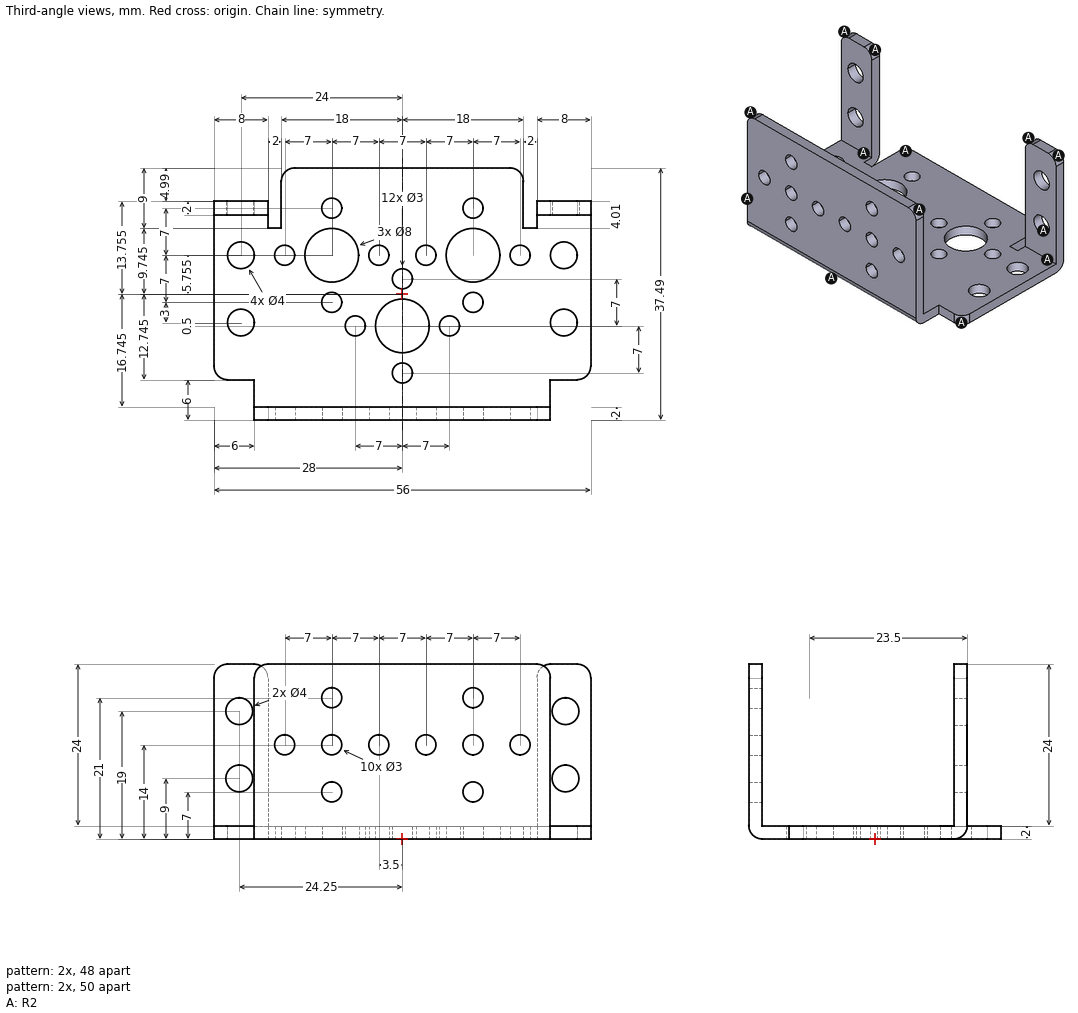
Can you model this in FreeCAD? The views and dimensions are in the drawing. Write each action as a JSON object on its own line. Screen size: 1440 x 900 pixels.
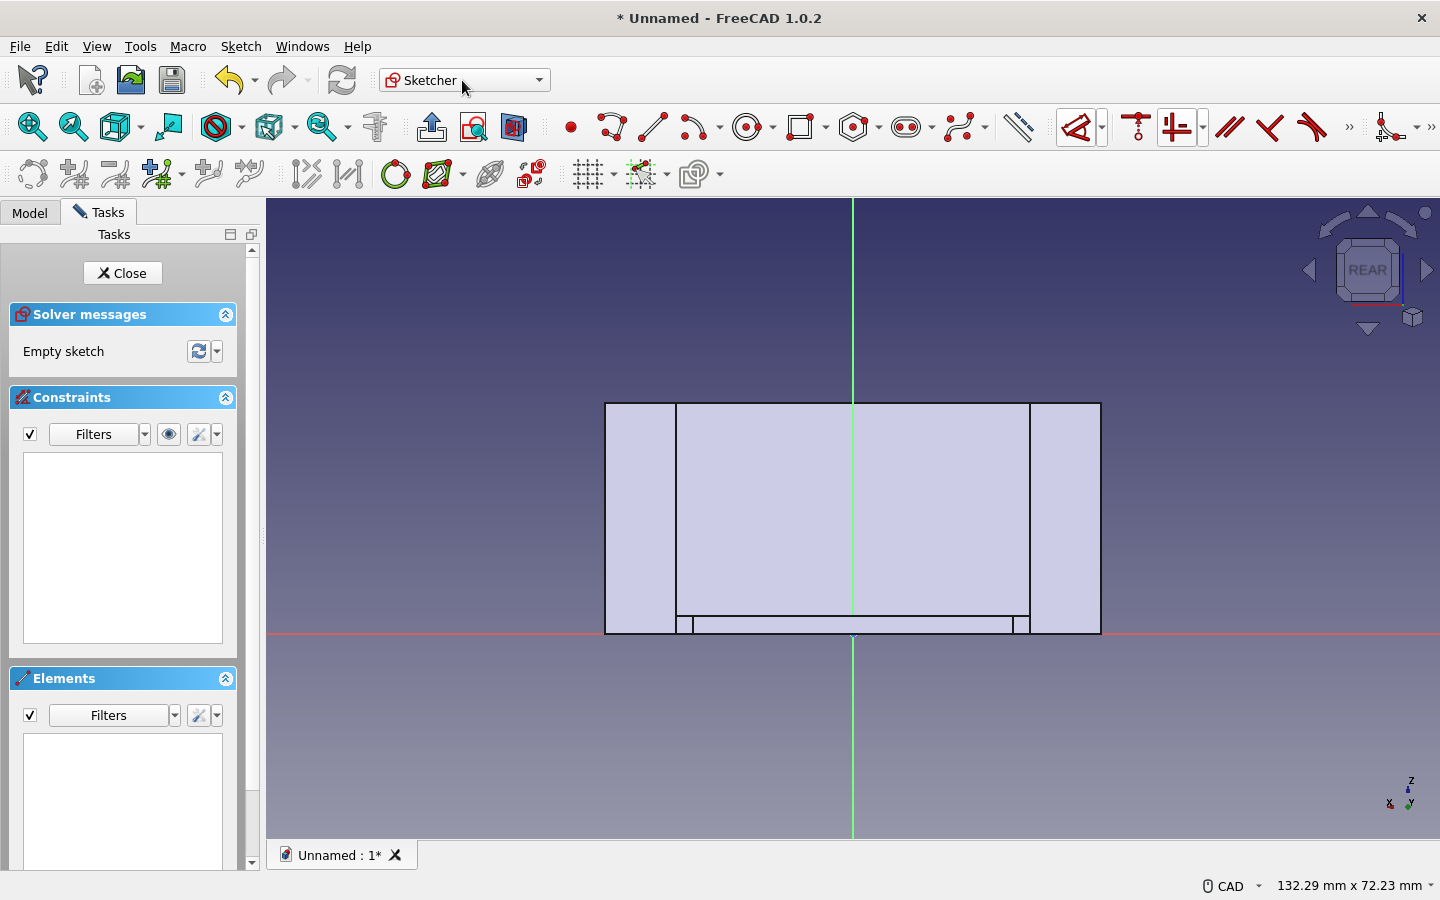
{"action": "key", "text": "q s"}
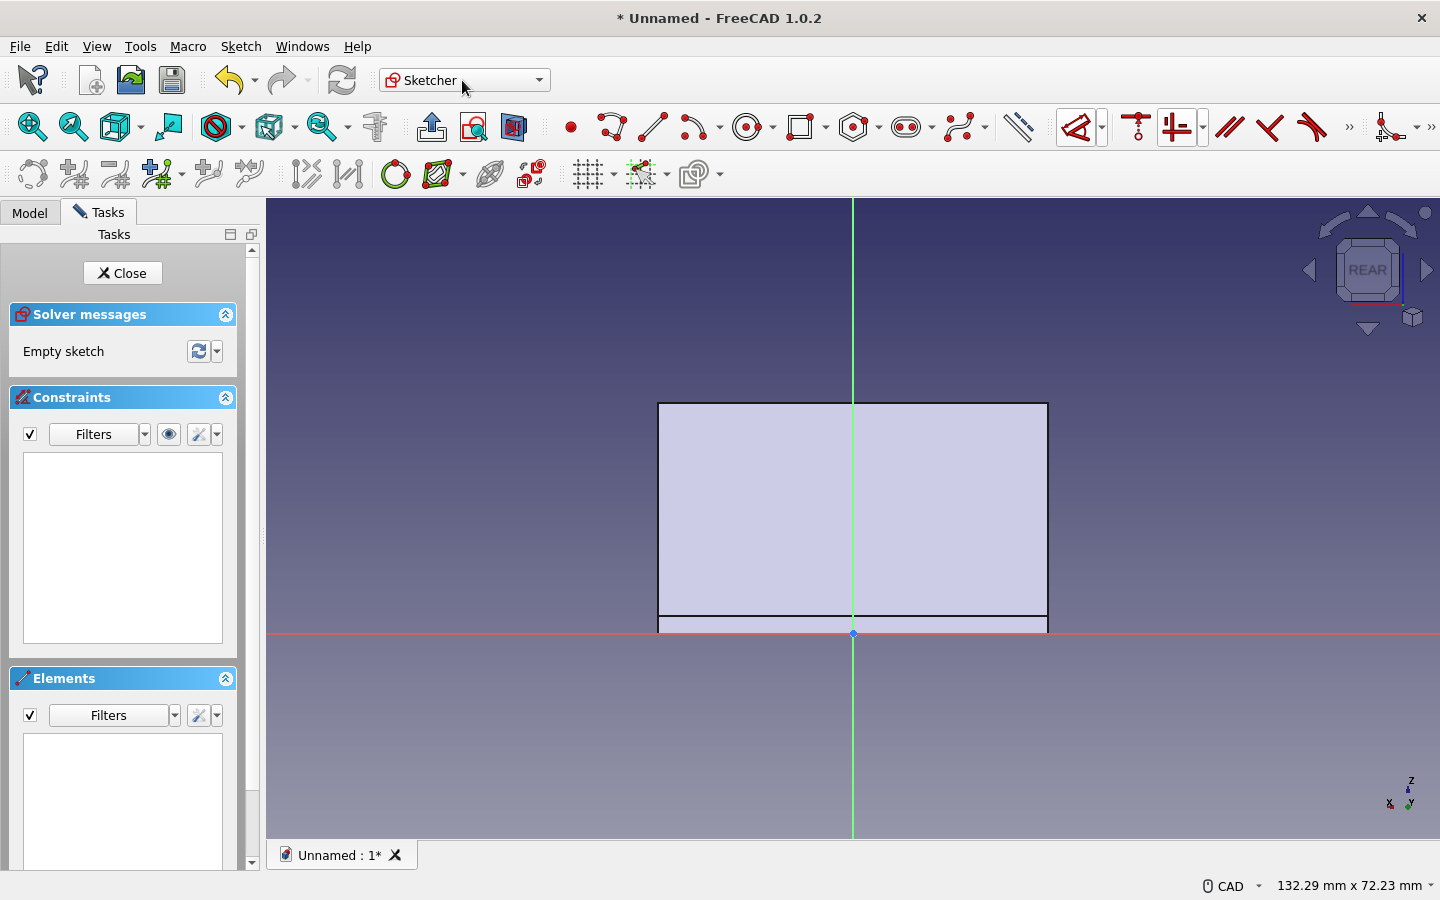
{"action": "scroll", "coordinate": [909, 547], "scroll_direction": "up", "scroll_amount": 4}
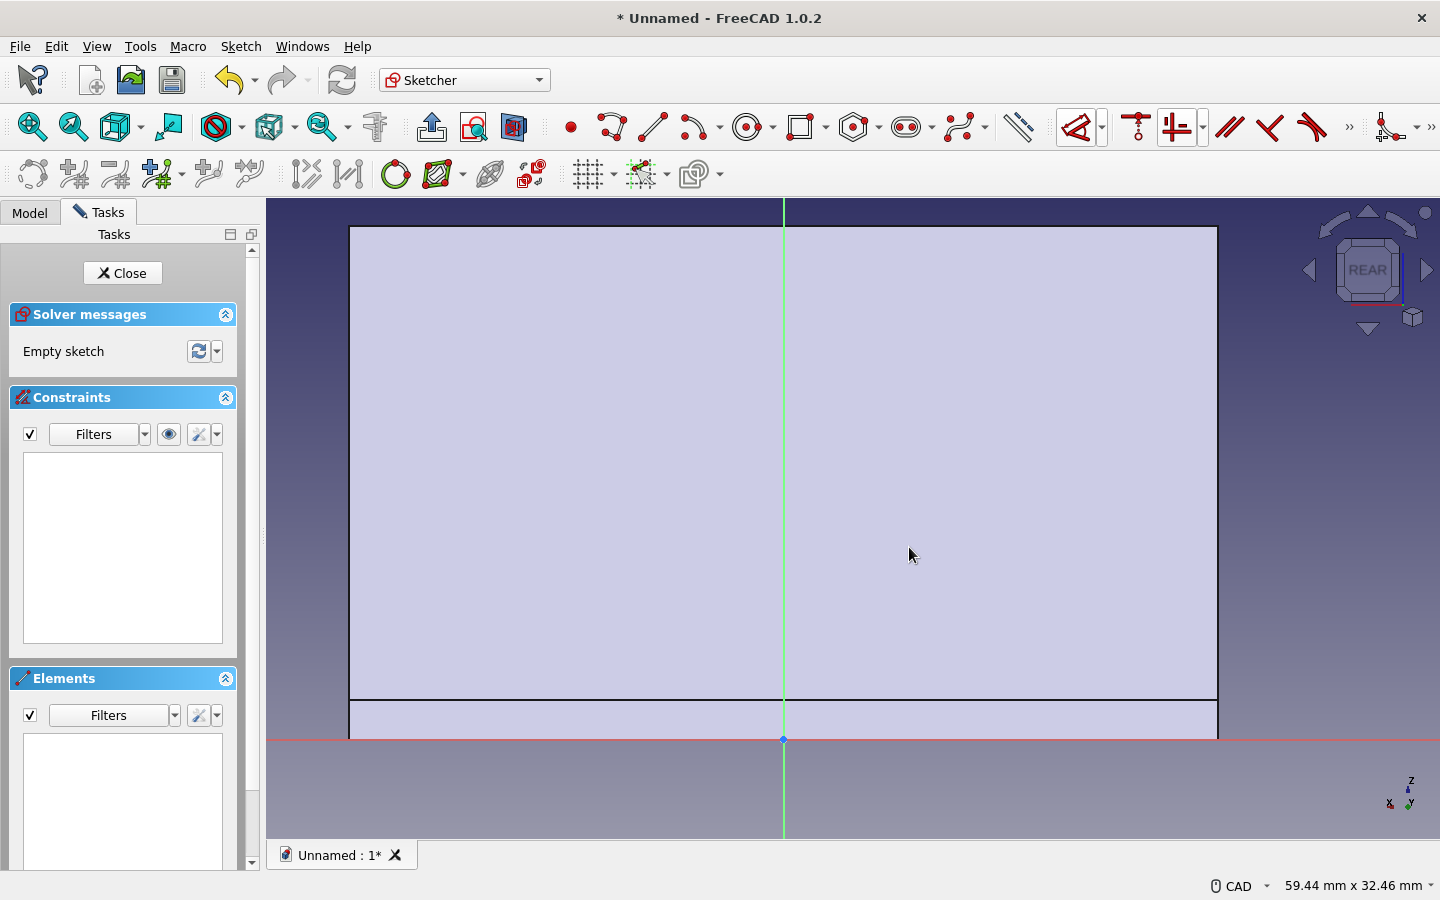
{"action": "key", "text": "g c"}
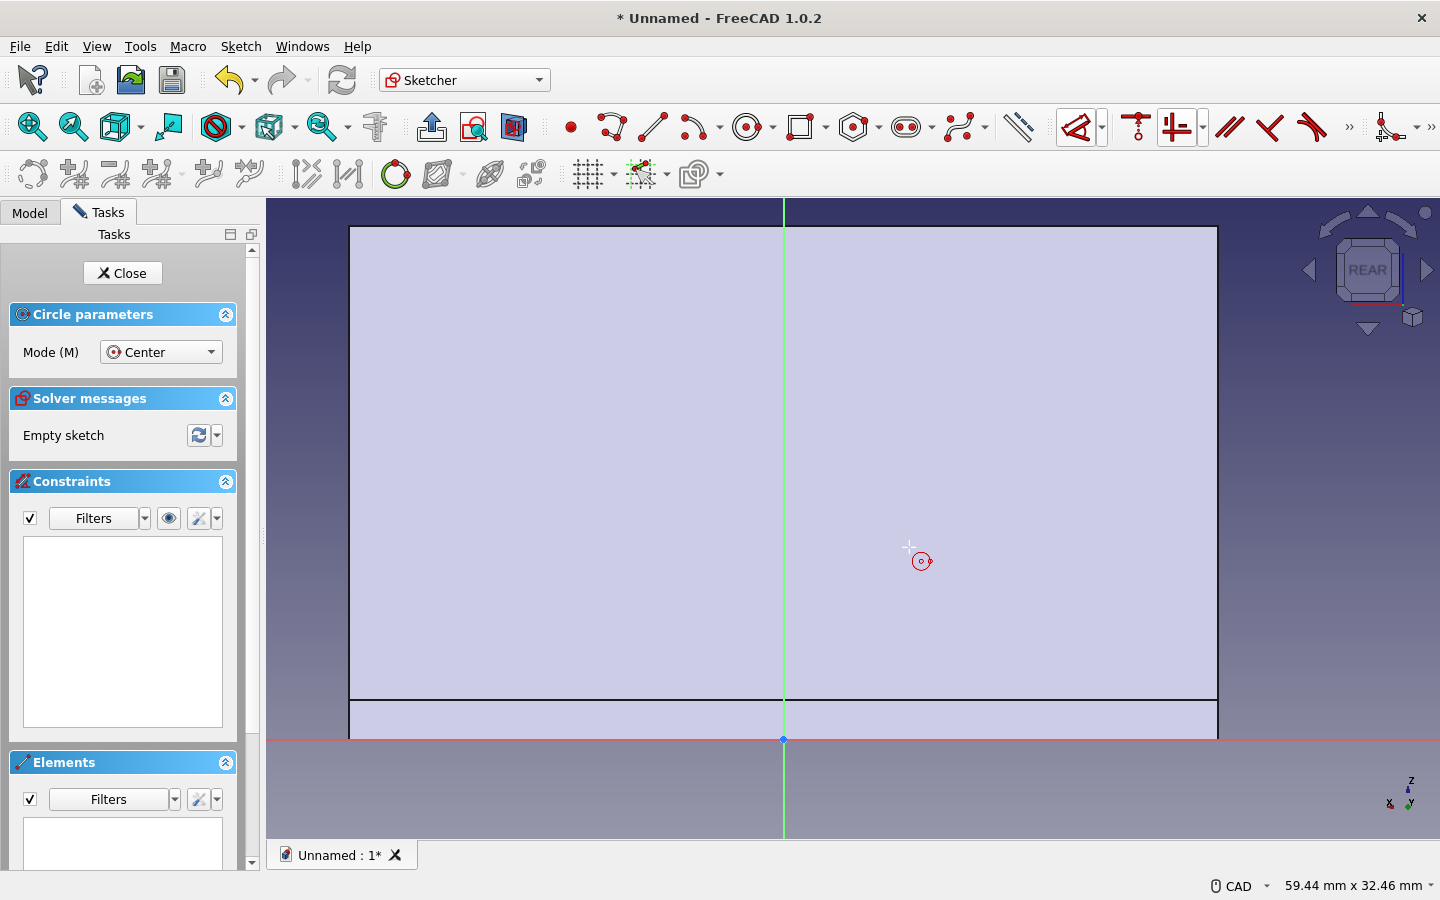
{"action": "left_click", "coordinate": [991, 463]}
{"action": "mouse_move", "coordinate": [1012, 442]}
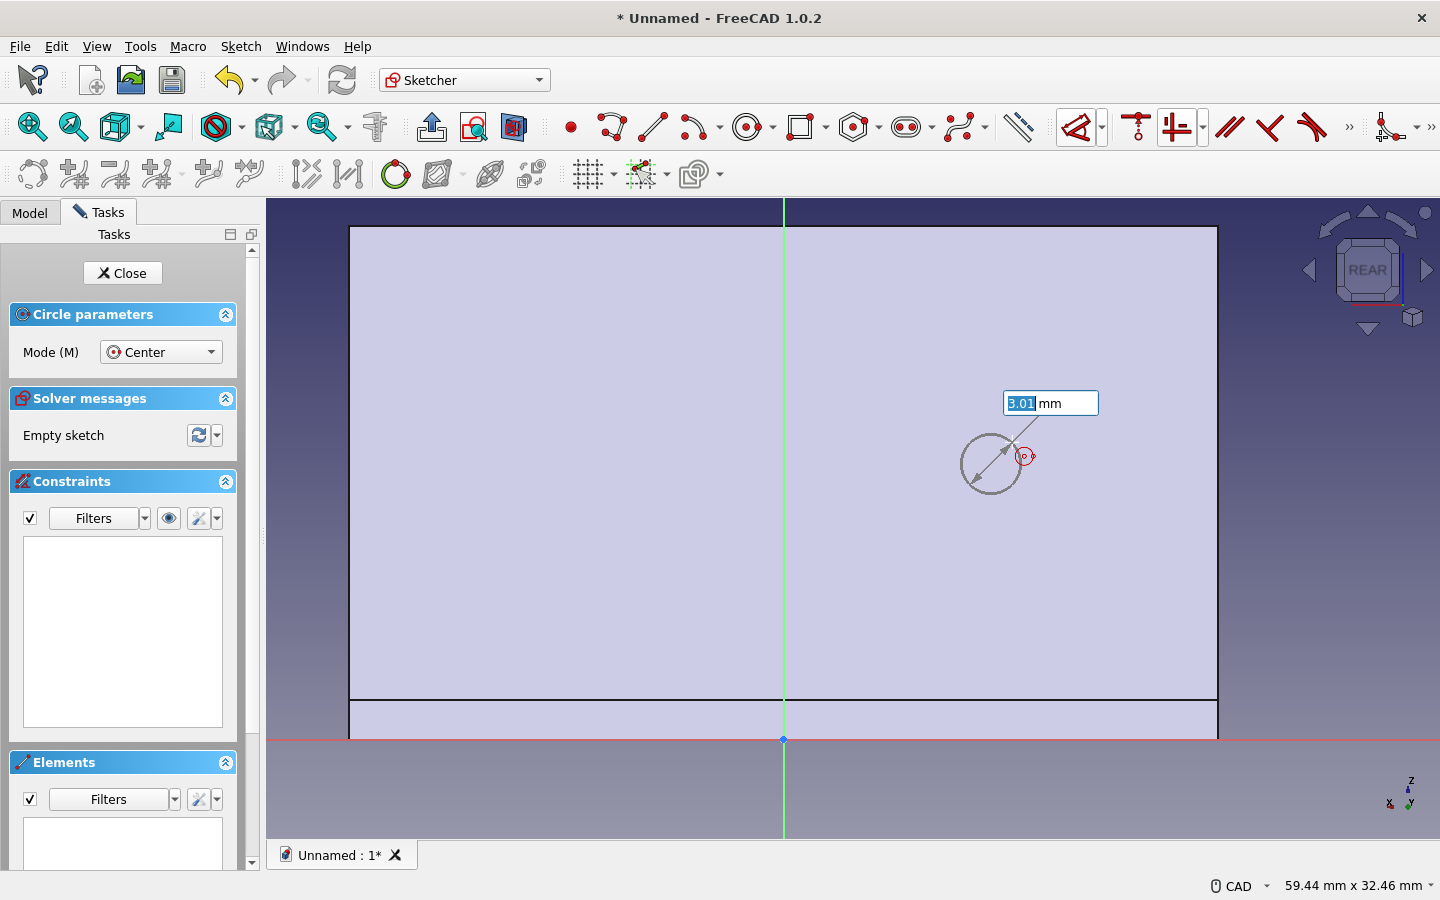
{"action": "type", "text": "3"}
{"action": "key", "text": "Return"}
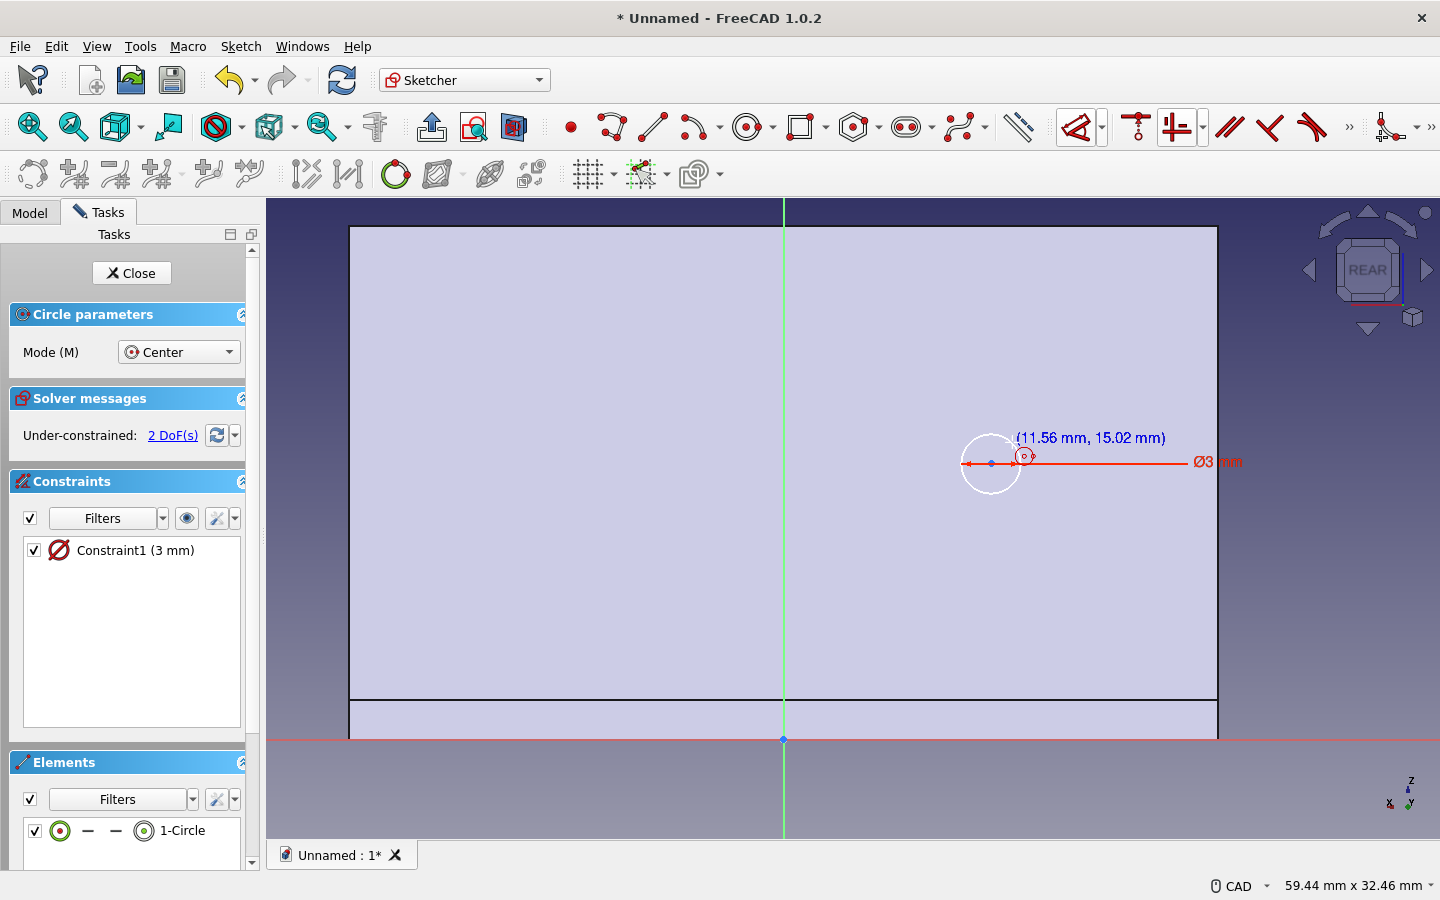
{"action": "left_click", "coordinate": [1129, 463]}
{"action": "mouse_move", "coordinate": [1150, 442]}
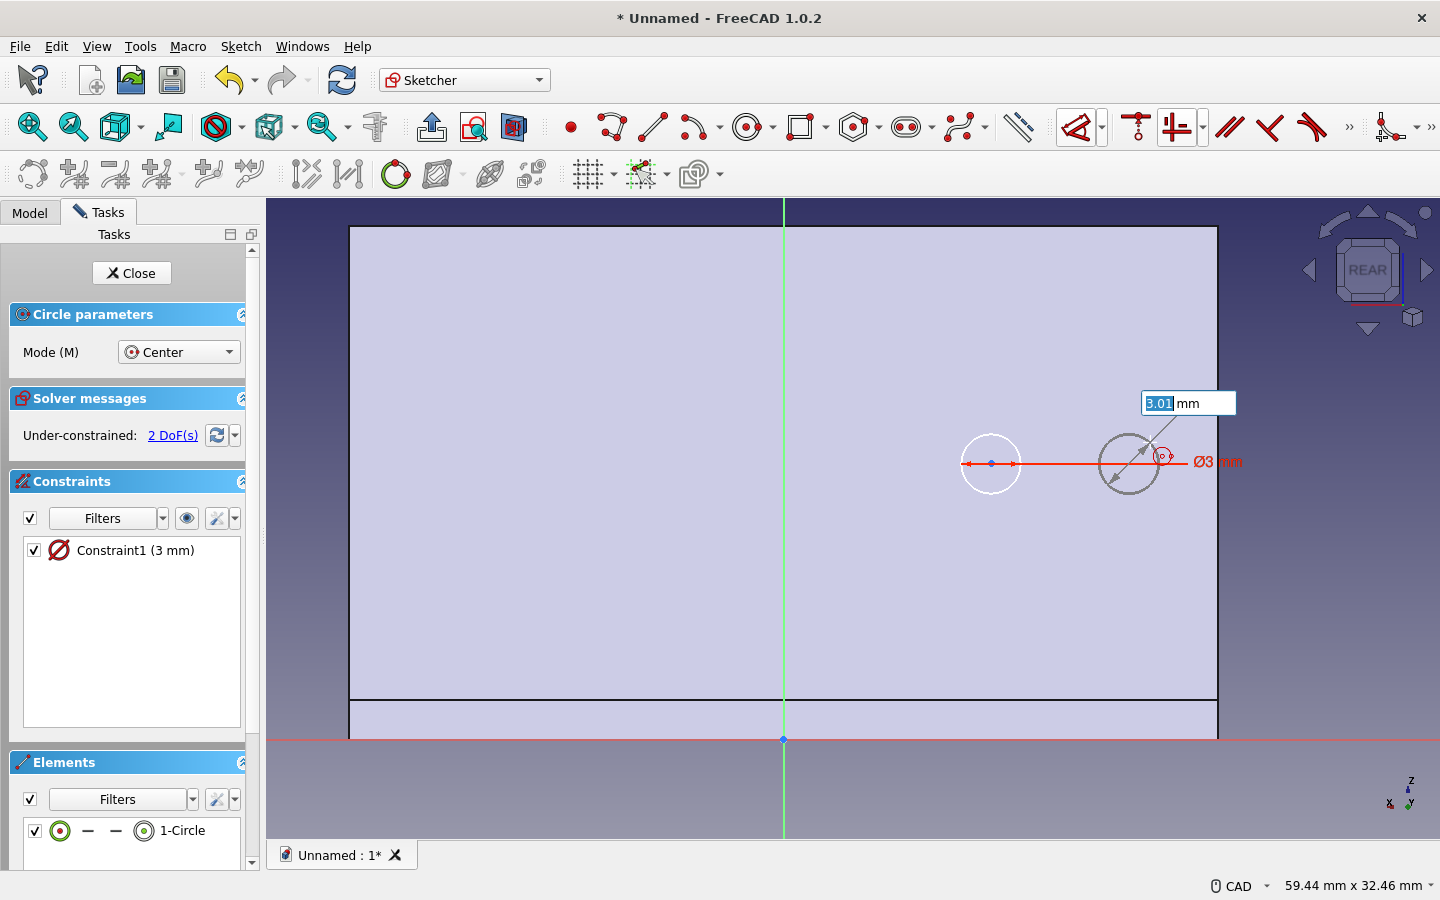
{"action": "type", "text": "3"}
{"action": "key", "text": "Return"}